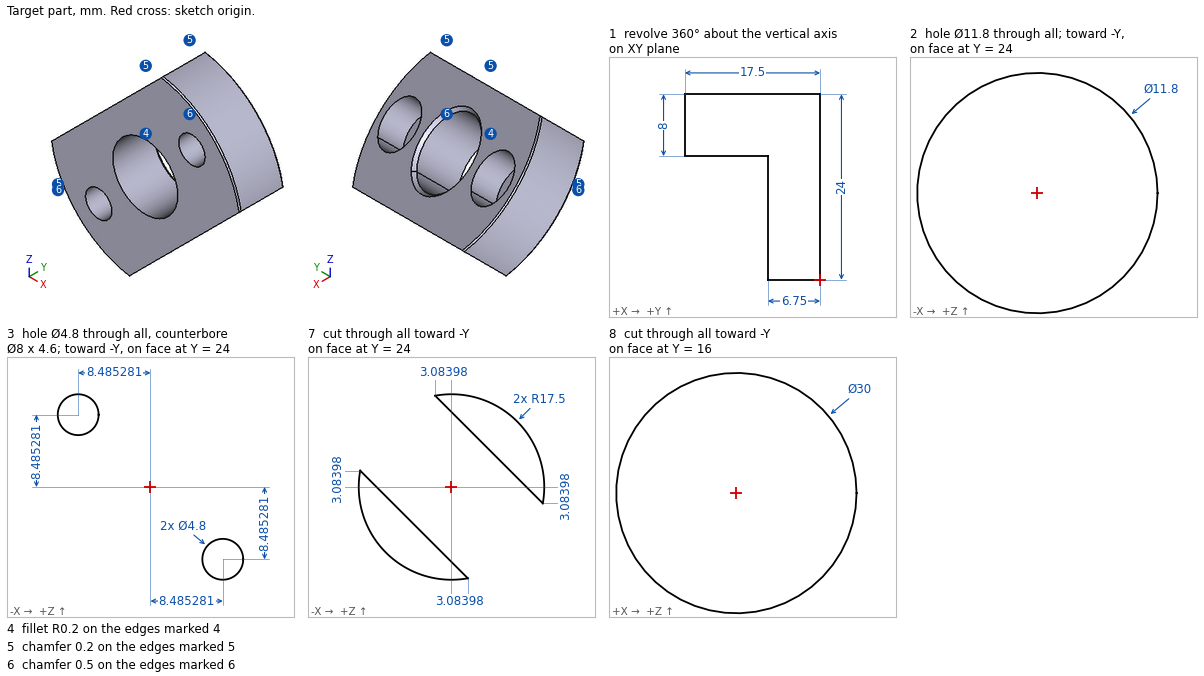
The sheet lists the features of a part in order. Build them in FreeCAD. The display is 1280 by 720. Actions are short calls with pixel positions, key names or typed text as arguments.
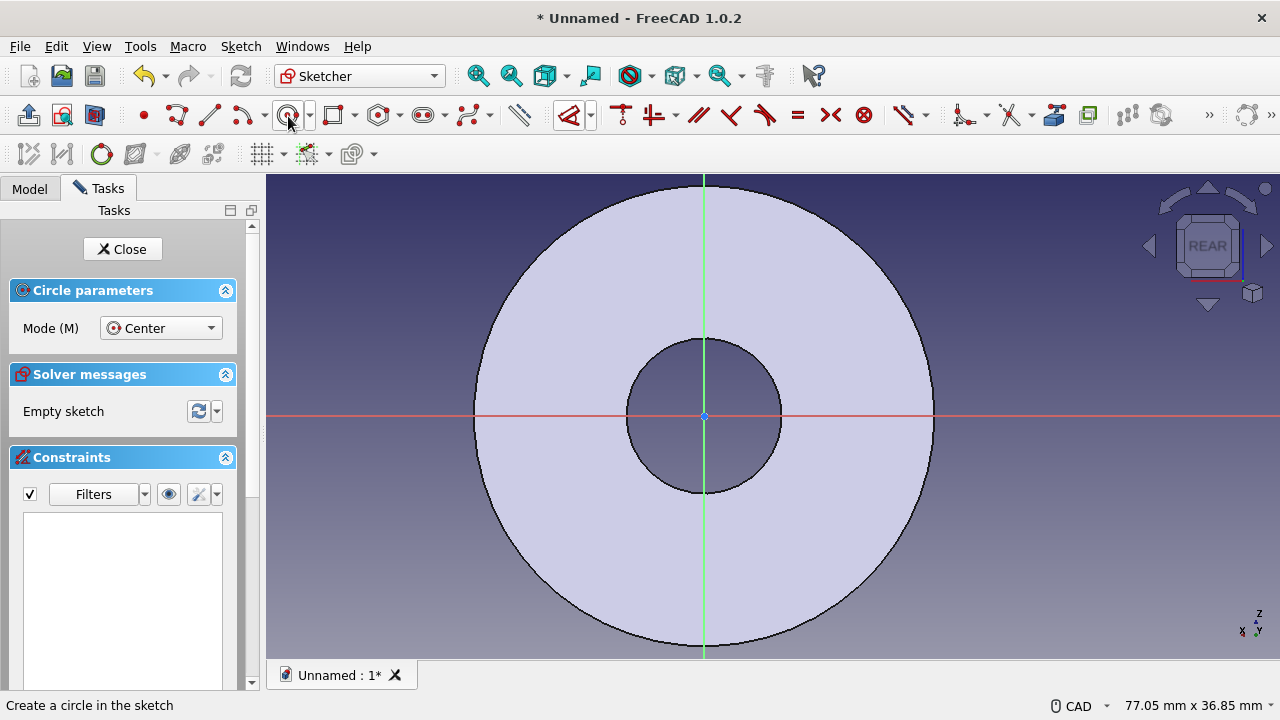
click(816, 528)
move(838, 505)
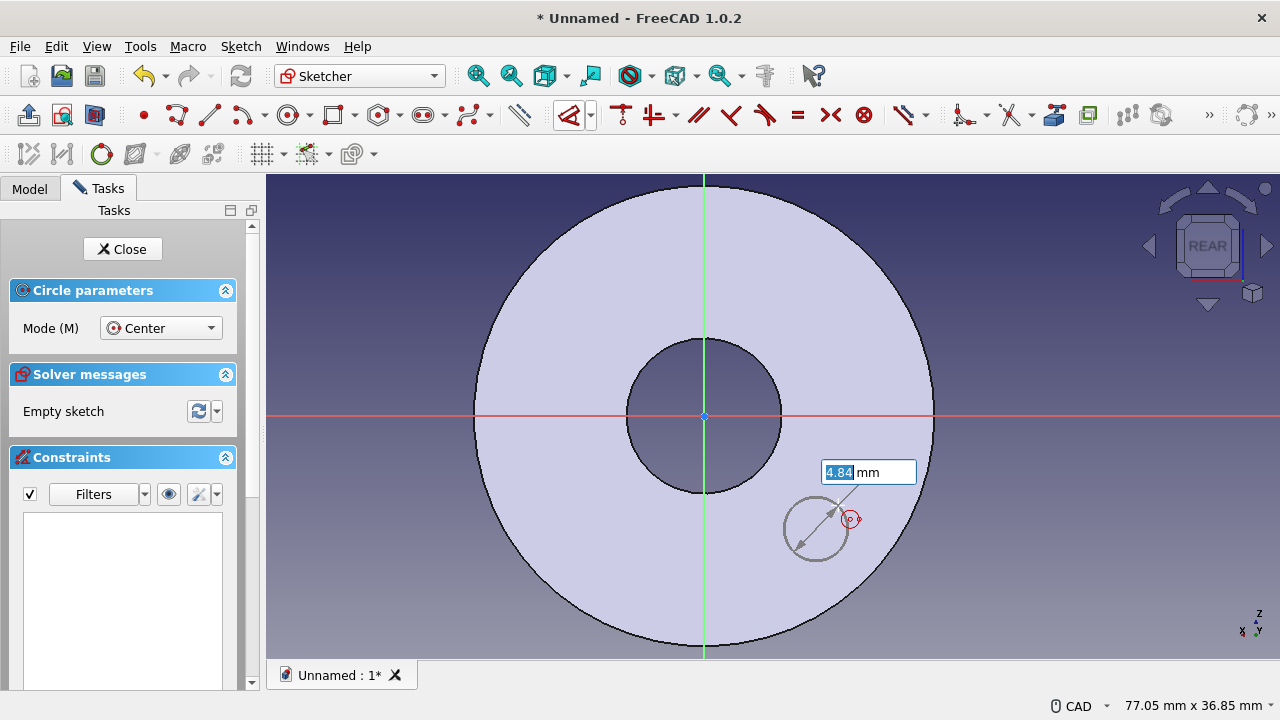
text(4.8)
key(Return)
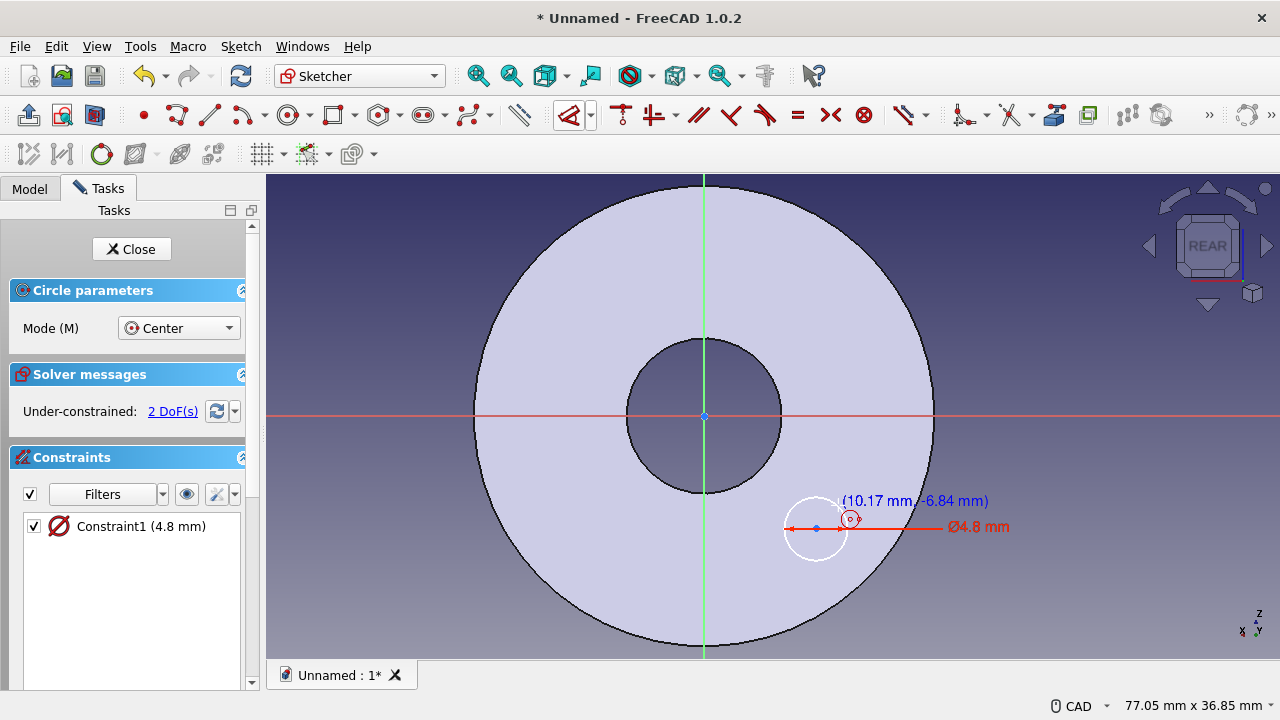
click(592, 304)
move(615, 282)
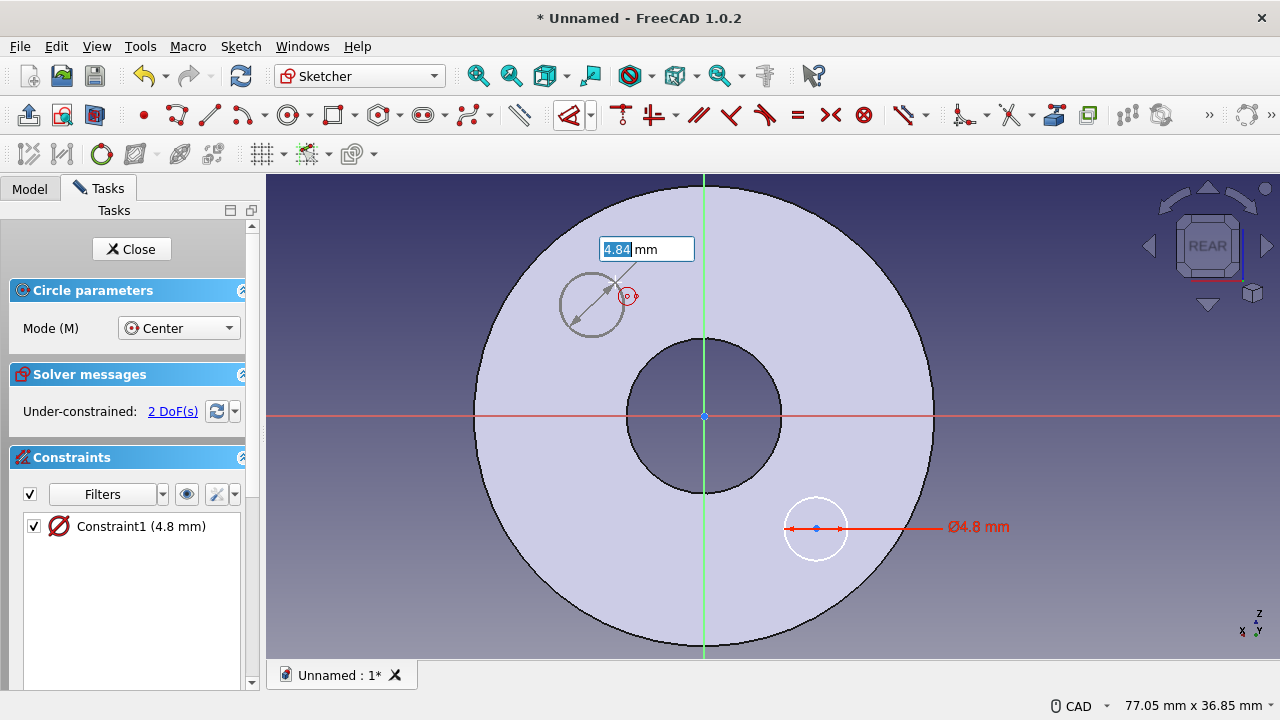
text(4.8)
key(Return)
key(Escape)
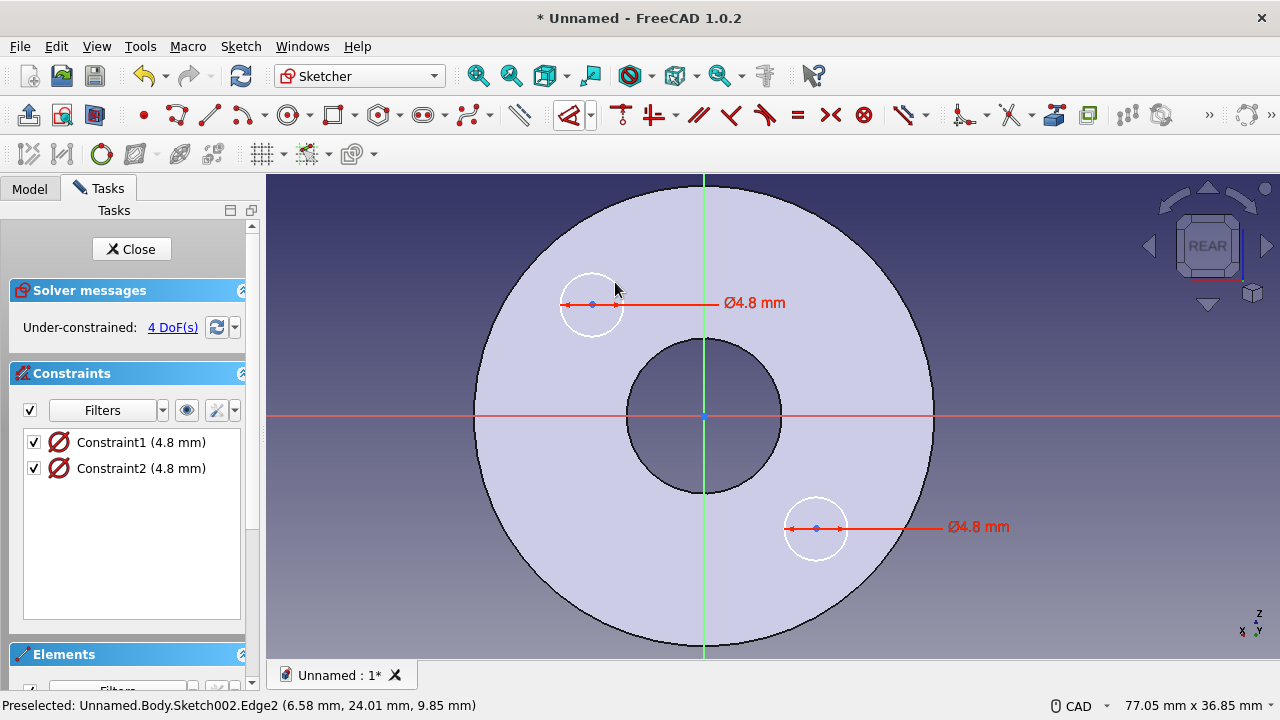
click(816, 529)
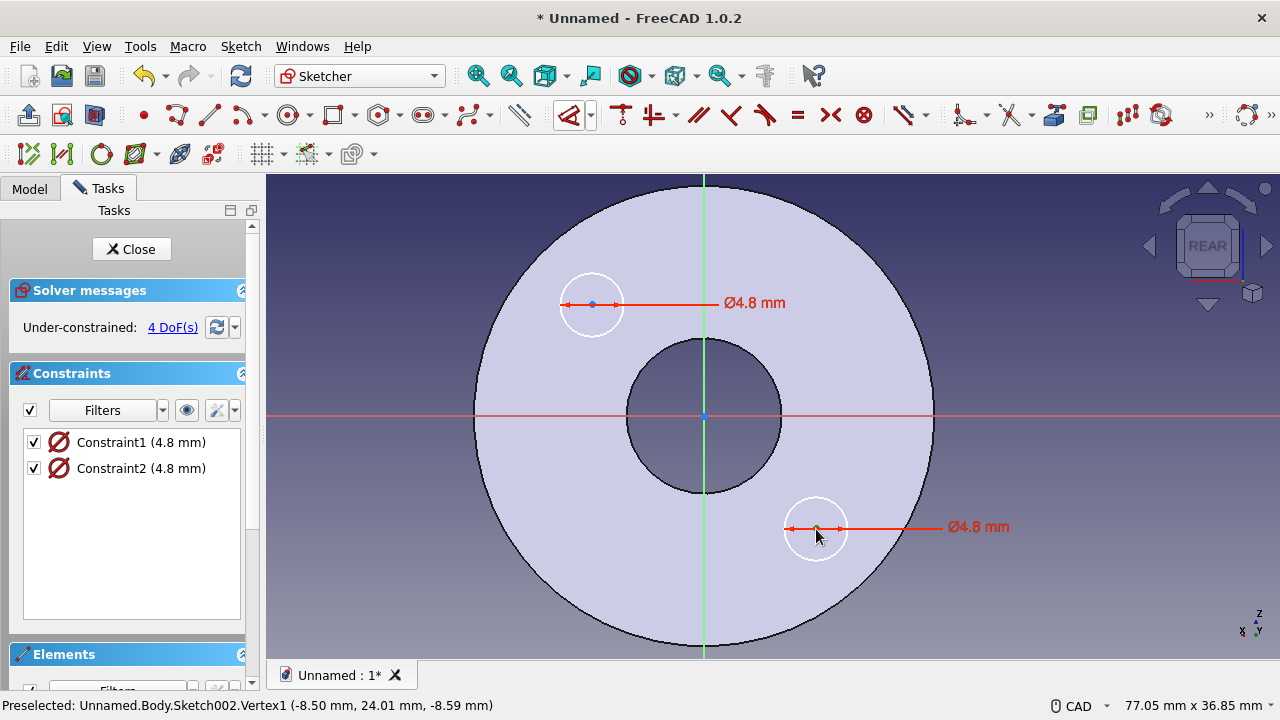
click(590, 116)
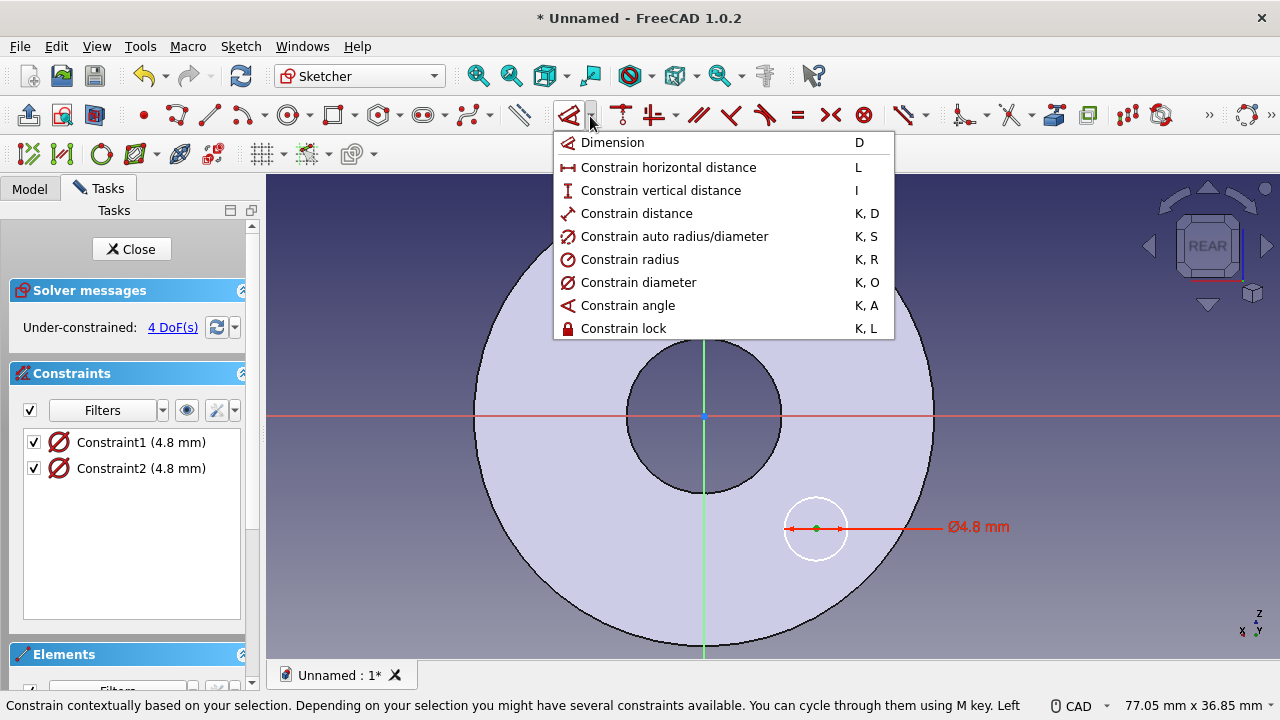
click(724, 168)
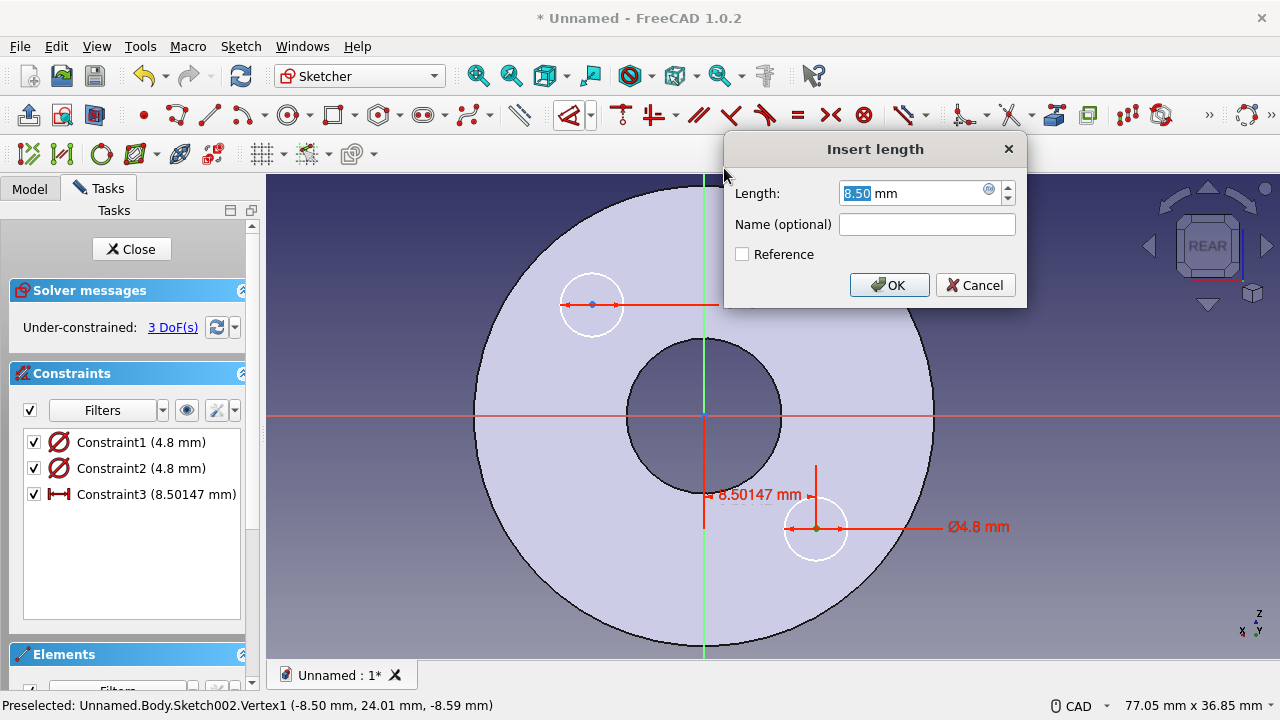
text(8.485281)
key(Return)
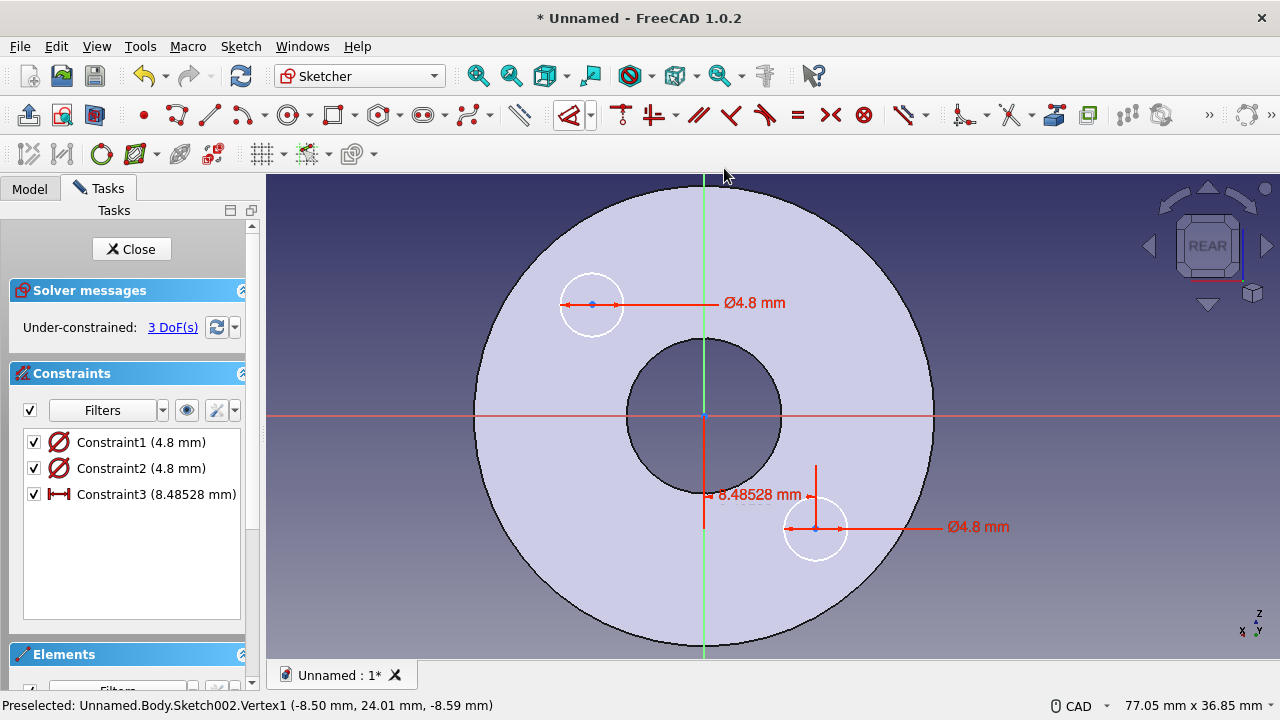
click(816, 529)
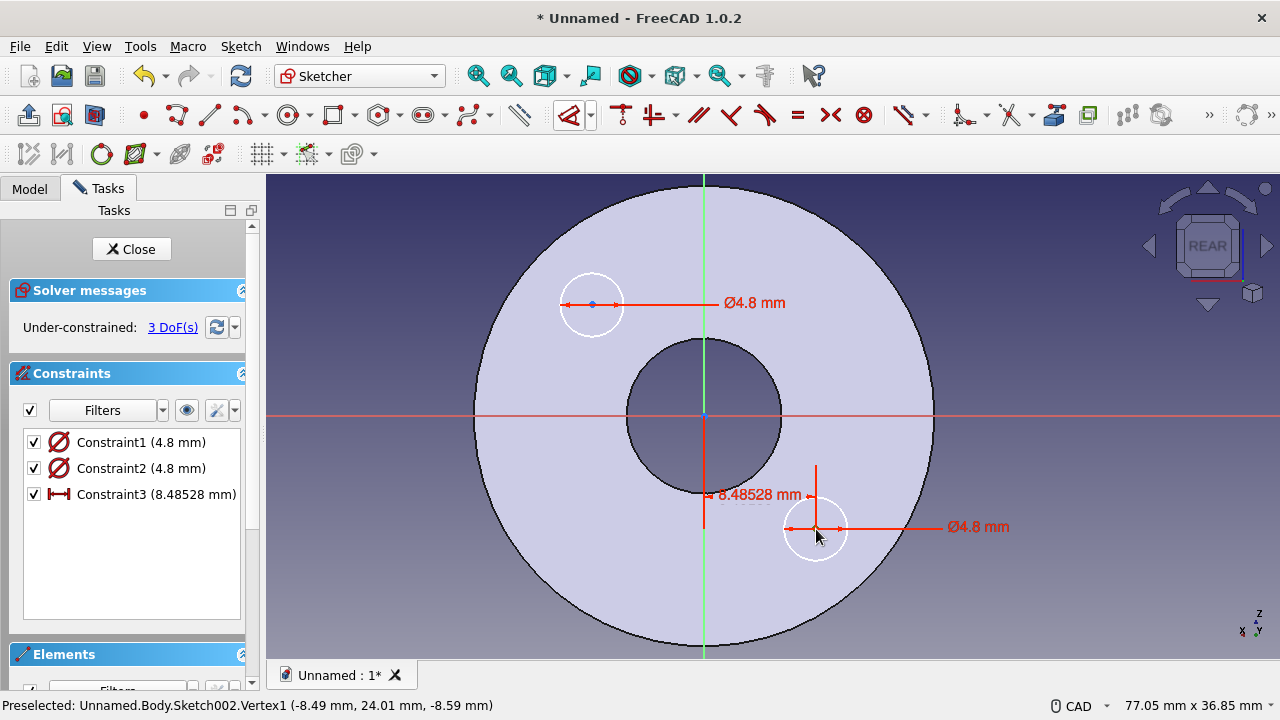
click(590, 116)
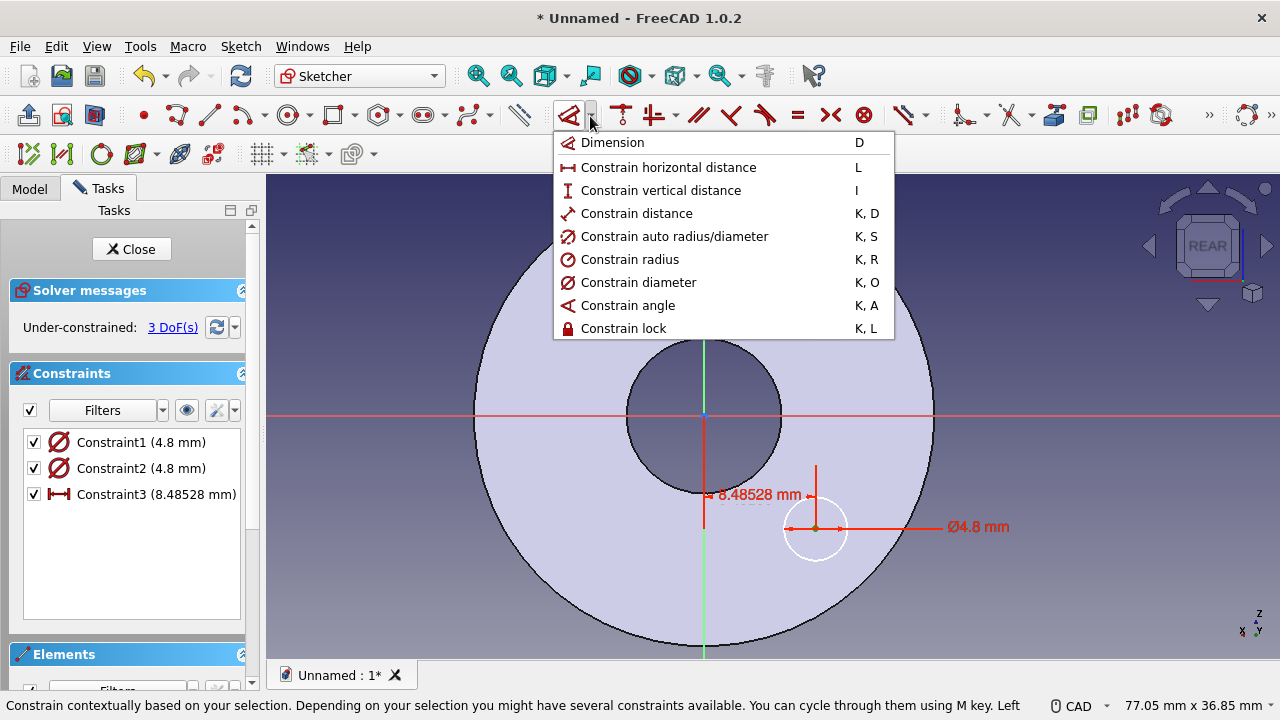
click(724, 190)